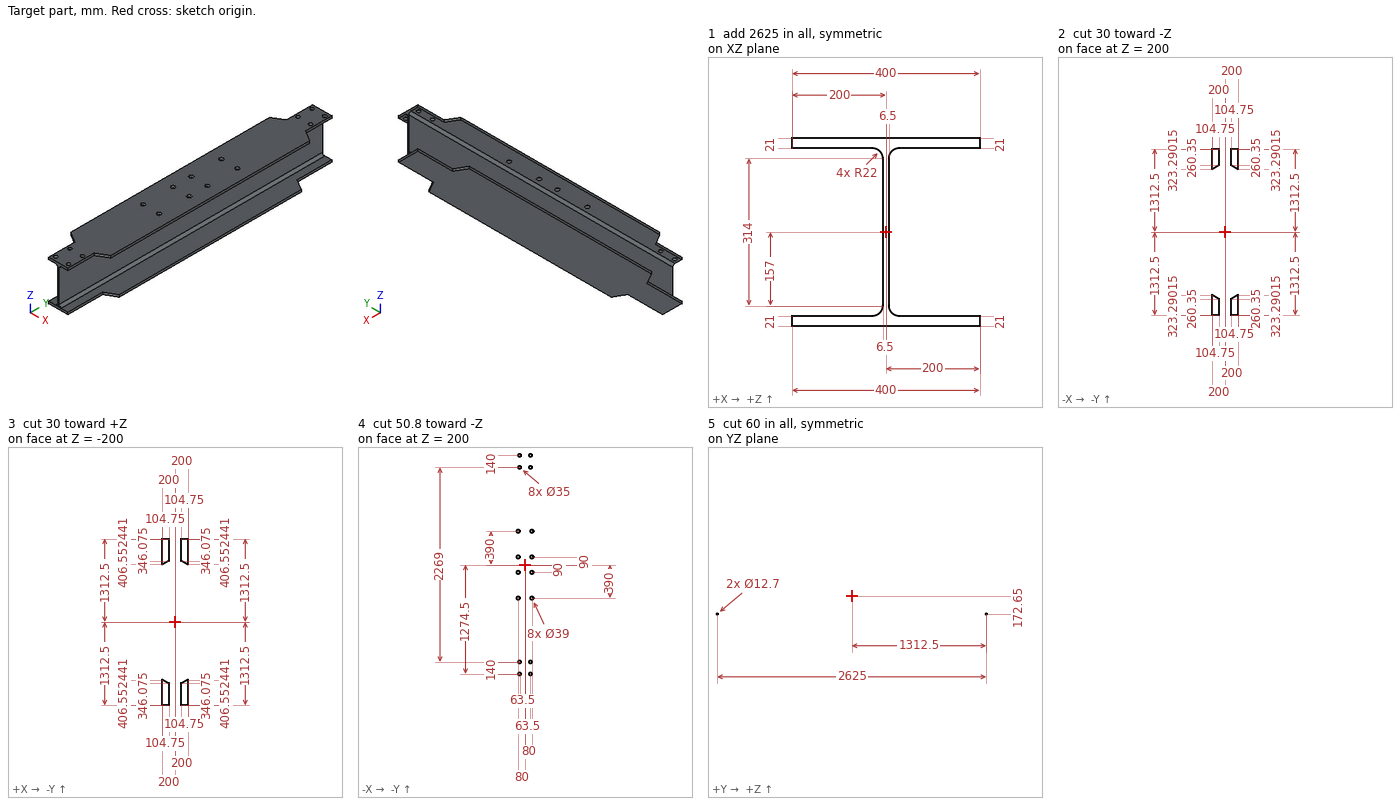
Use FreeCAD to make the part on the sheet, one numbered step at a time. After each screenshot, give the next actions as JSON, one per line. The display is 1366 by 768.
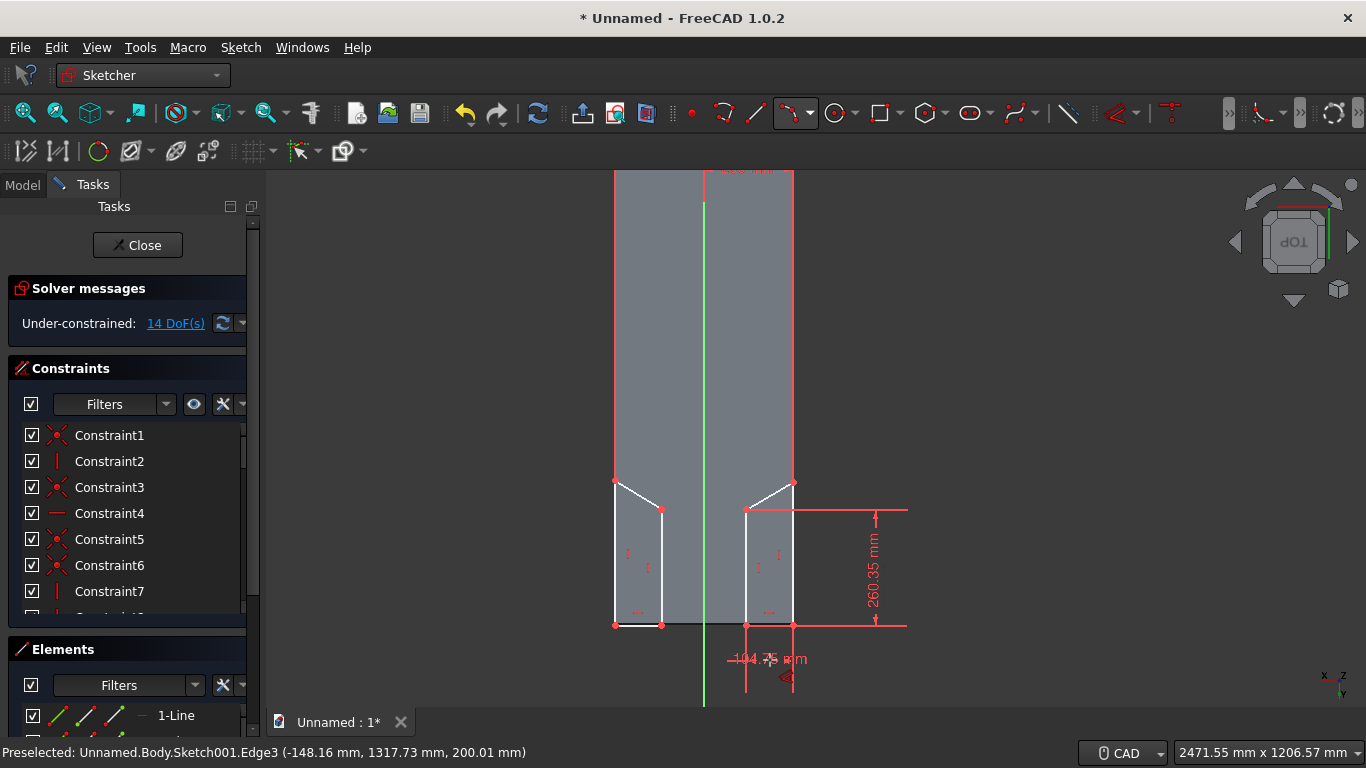
{"action": "left_click", "coordinate": [629, 626]}
{"action": "left_click", "coordinate": [638, 660]}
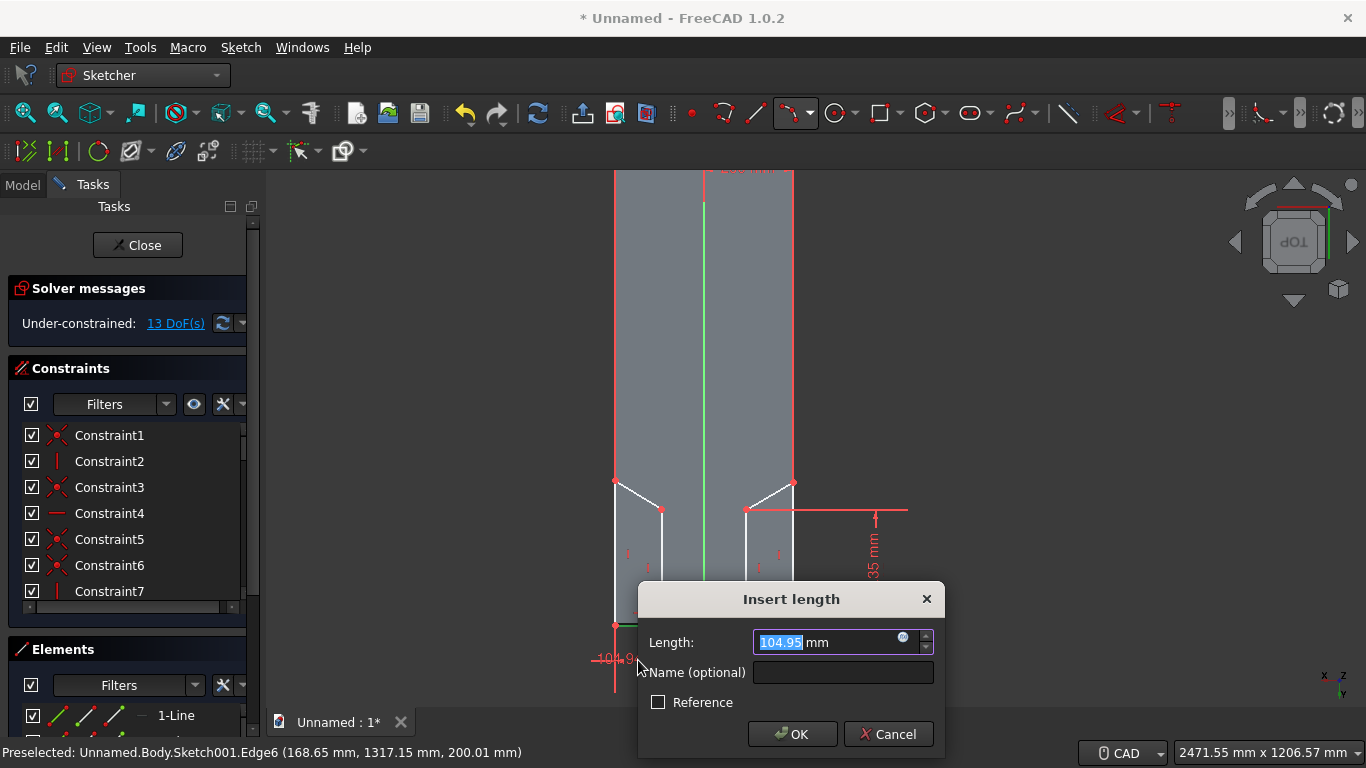
{"action": "type", "text": "104.75"}
{"action": "key", "text": "Return"}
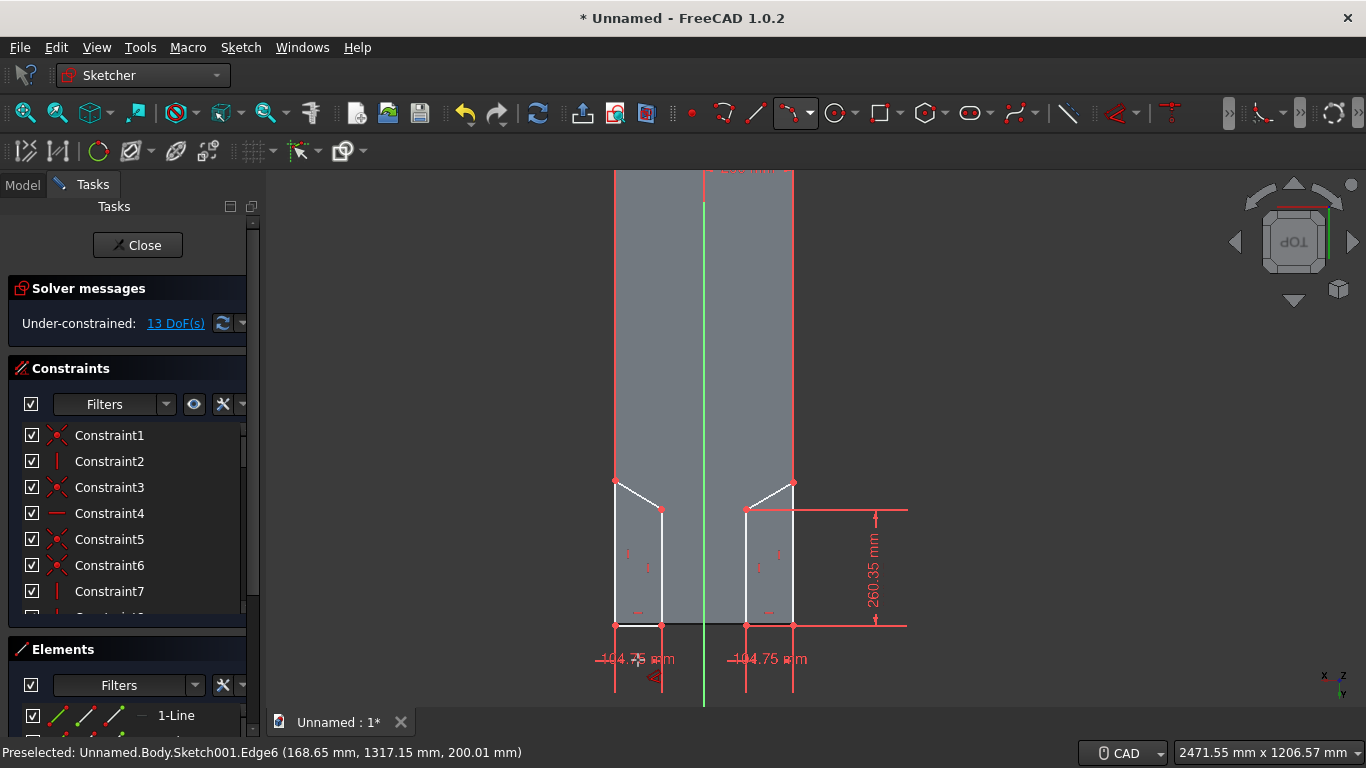
{"action": "left_click", "coordinate": [662, 591]}
{"action": "left_click", "coordinate": [720, 567]}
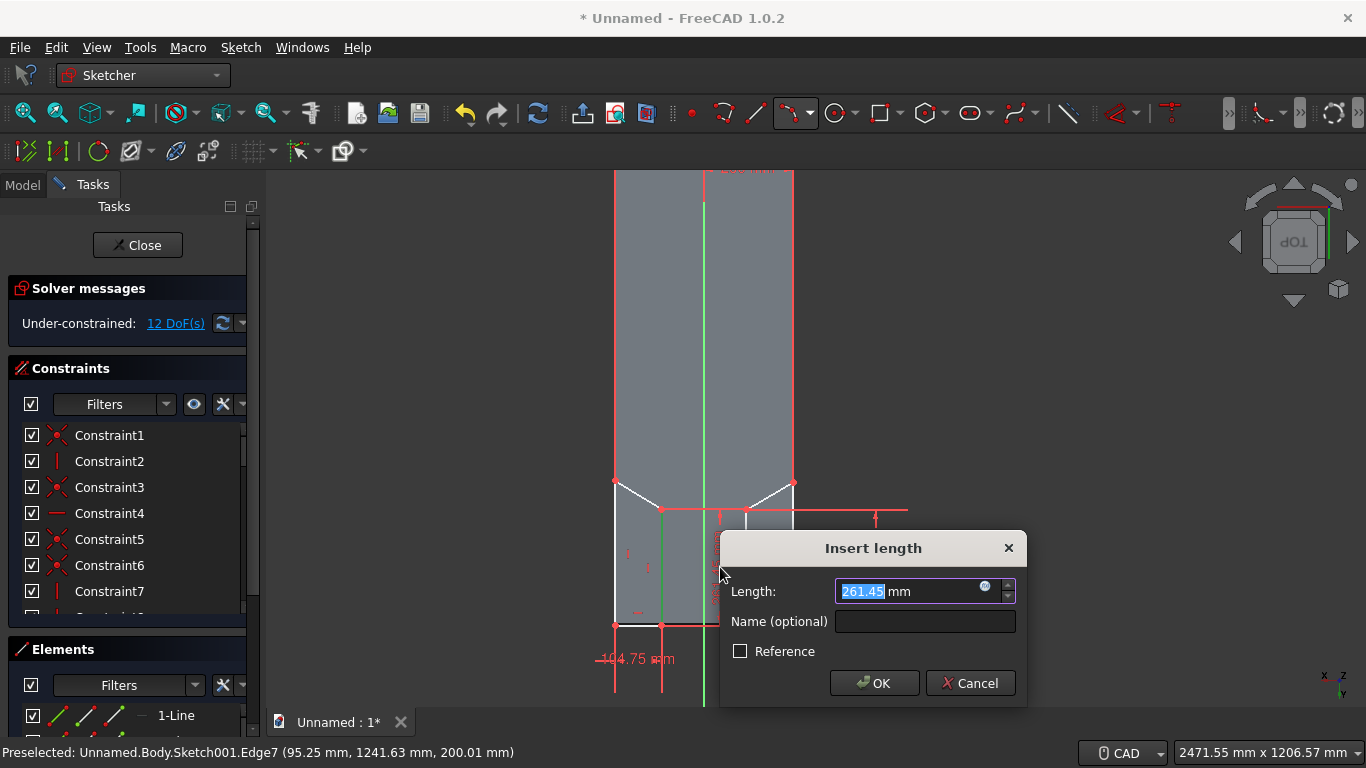
{"action": "type", "text": "260.35"}
{"action": "key", "text": "Return"}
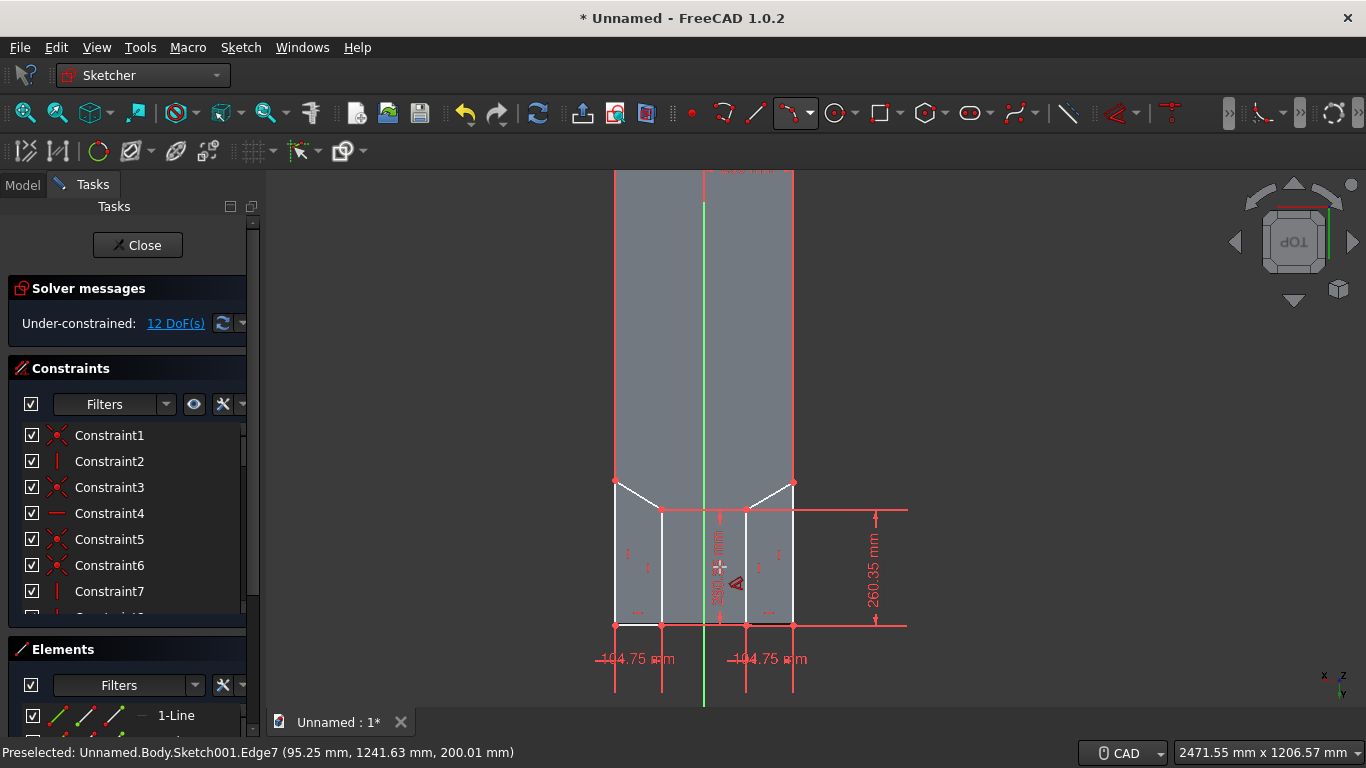
{"action": "scroll", "coordinate": [766, 611], "scroll_direction": "down", "scroll_amount": 6}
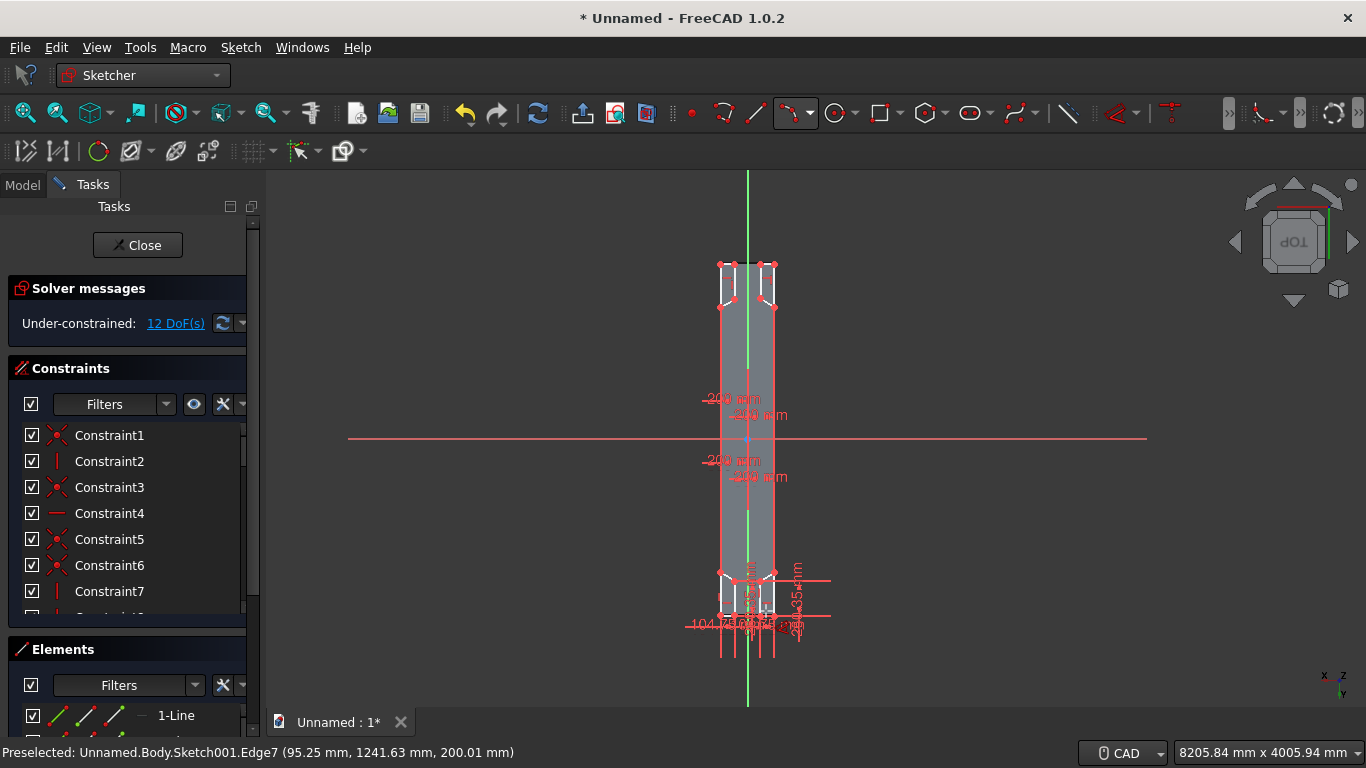
{"action": "scroll", "coordinate": [735, 289], "scroll_direction": "up", "scroll_amount": 2}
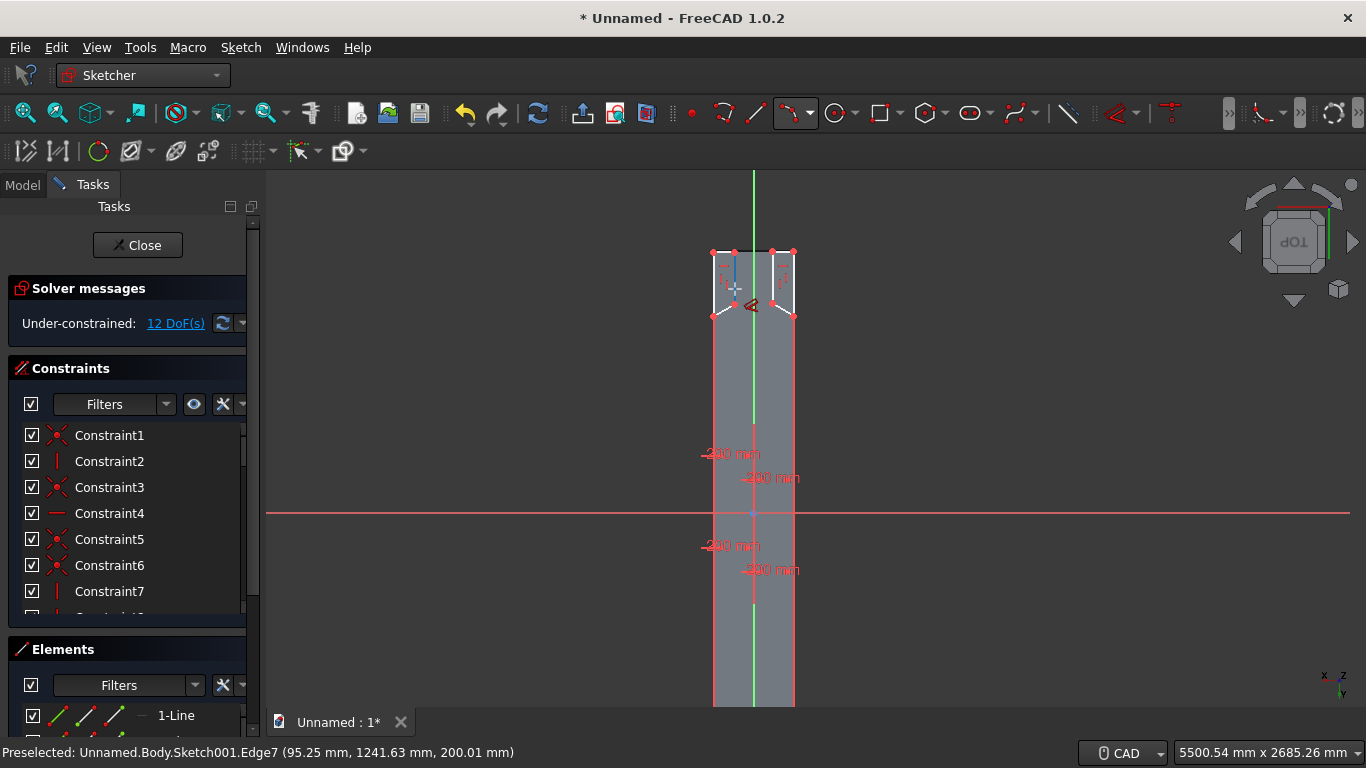
{"action": "left_click", "coordinate": [735, 289]}
{"action": "left_click", "coordinate": [677, 278]}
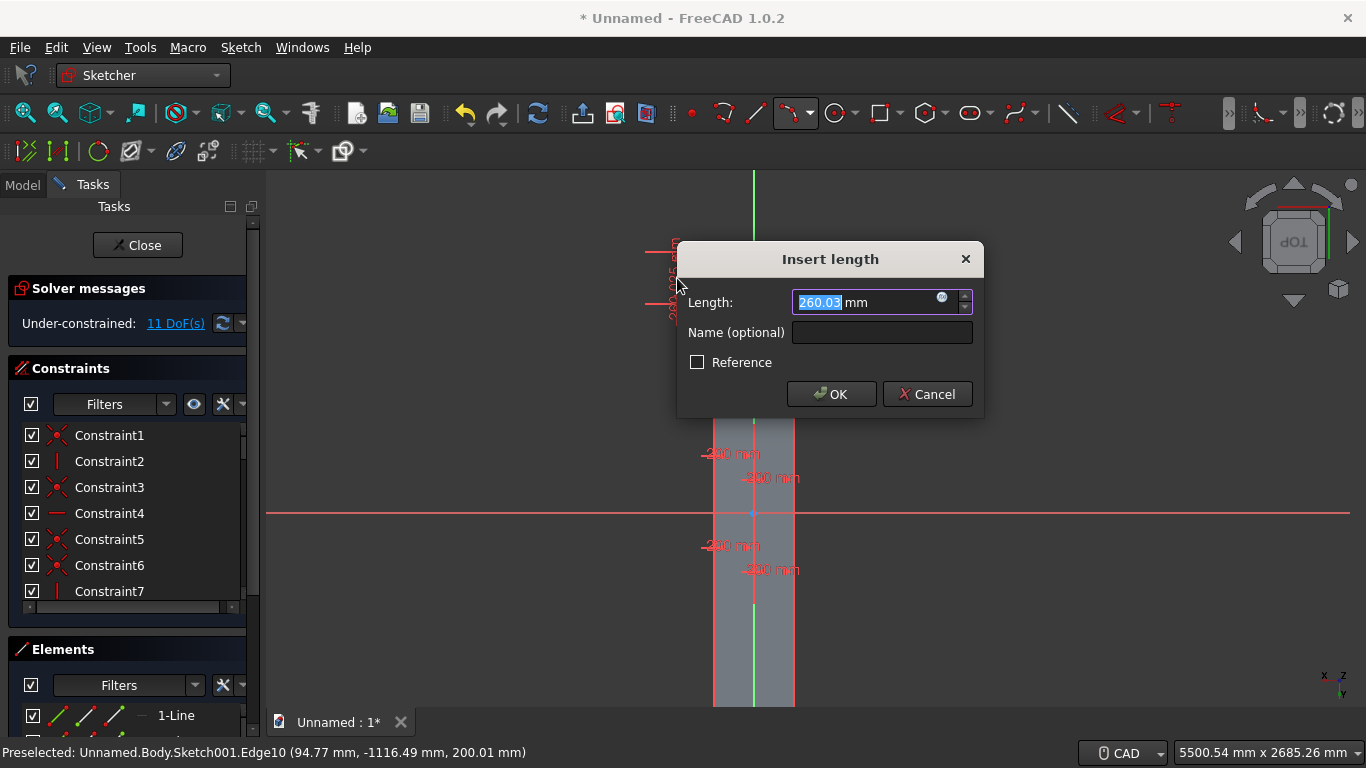
{"action": "type", "text": "260.35"}
{"action": "key", "text": "Return"}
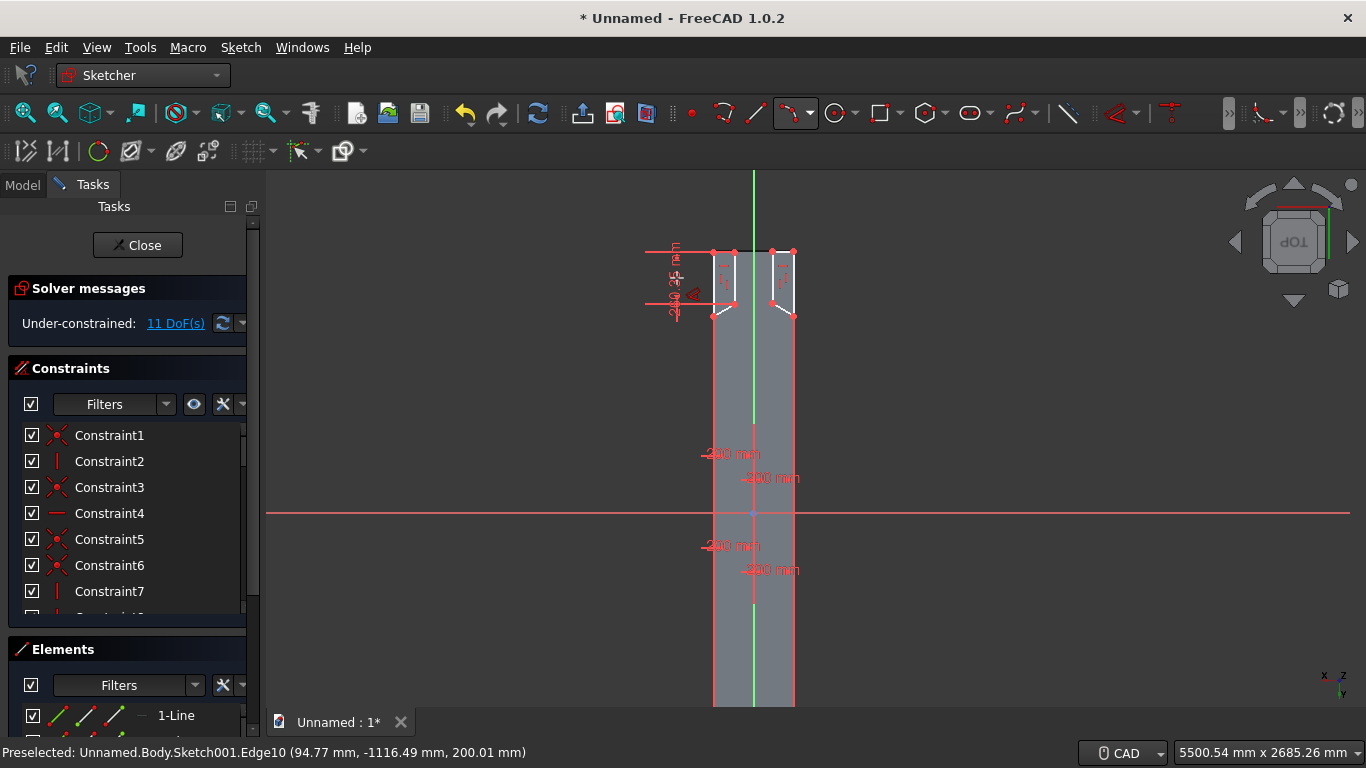
{"action": "scroll", "coordinate": [724, 252], "scroll_direction": "up", "scroll_amount": 4}